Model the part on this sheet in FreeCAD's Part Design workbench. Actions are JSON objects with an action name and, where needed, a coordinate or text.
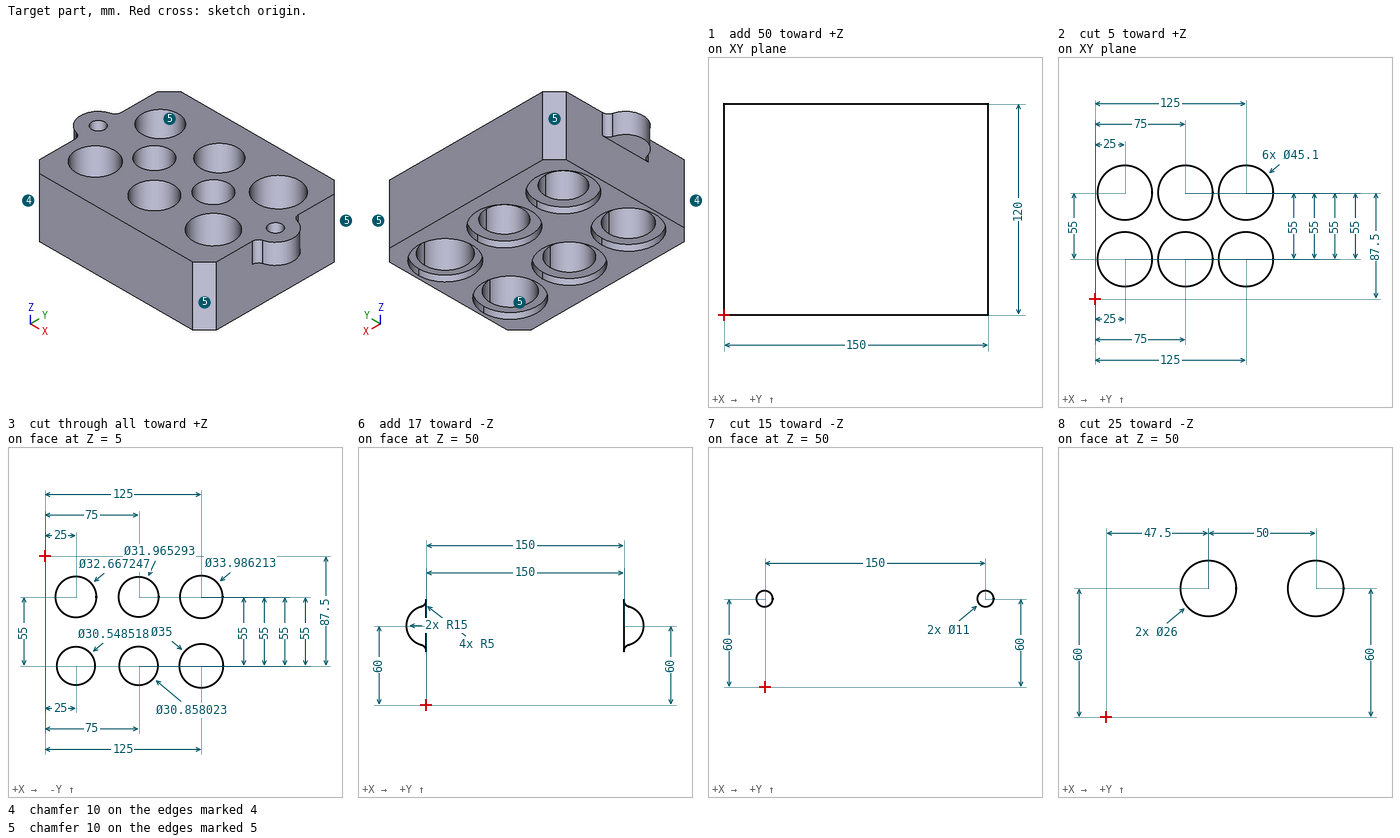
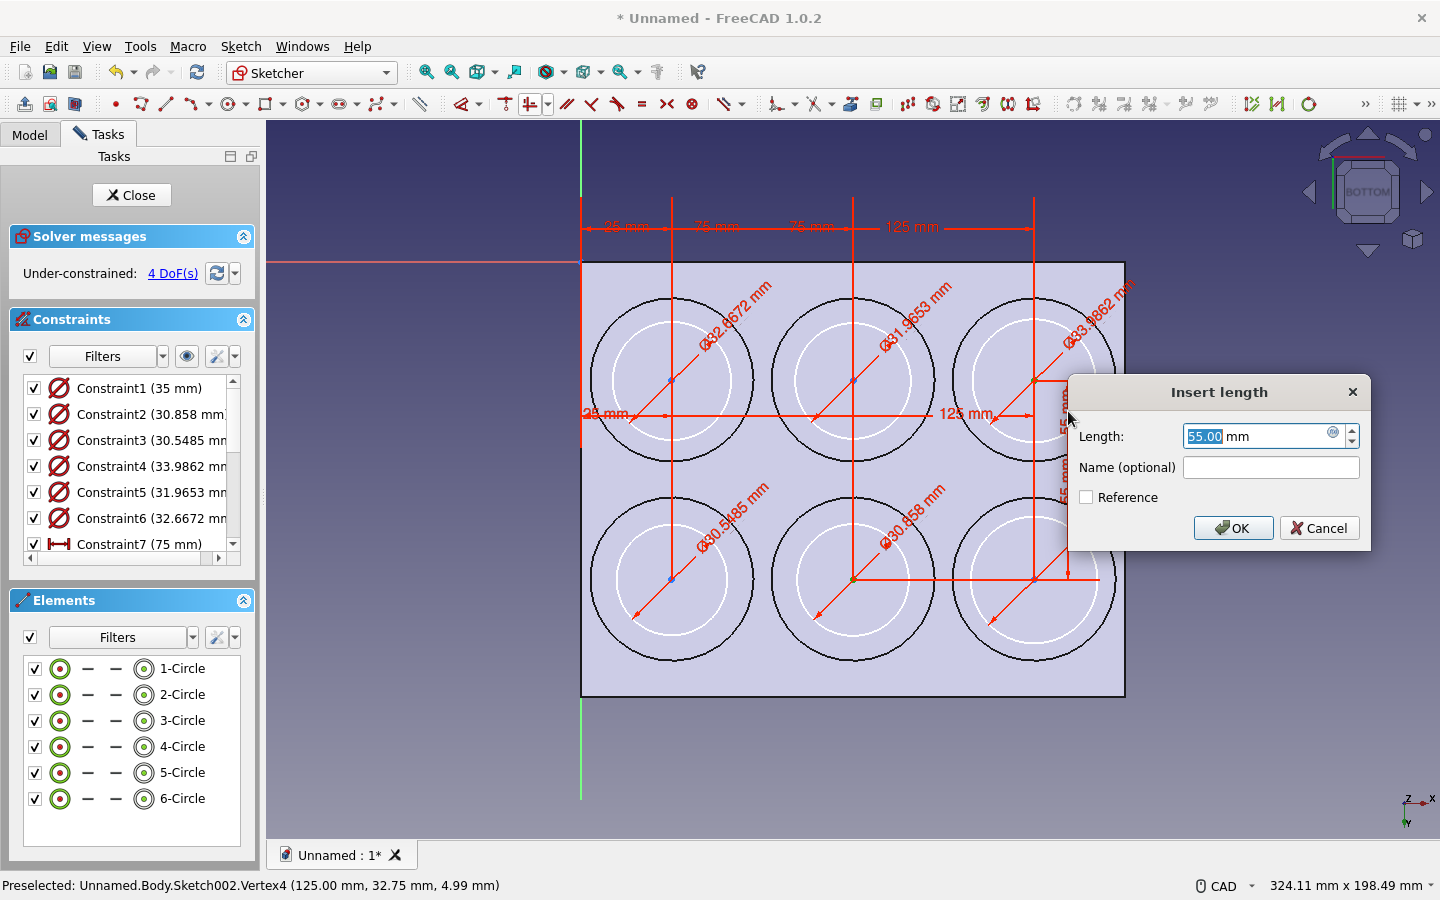
{"action": "type", "text": "55"}
{"action": "key", "text": "Return"}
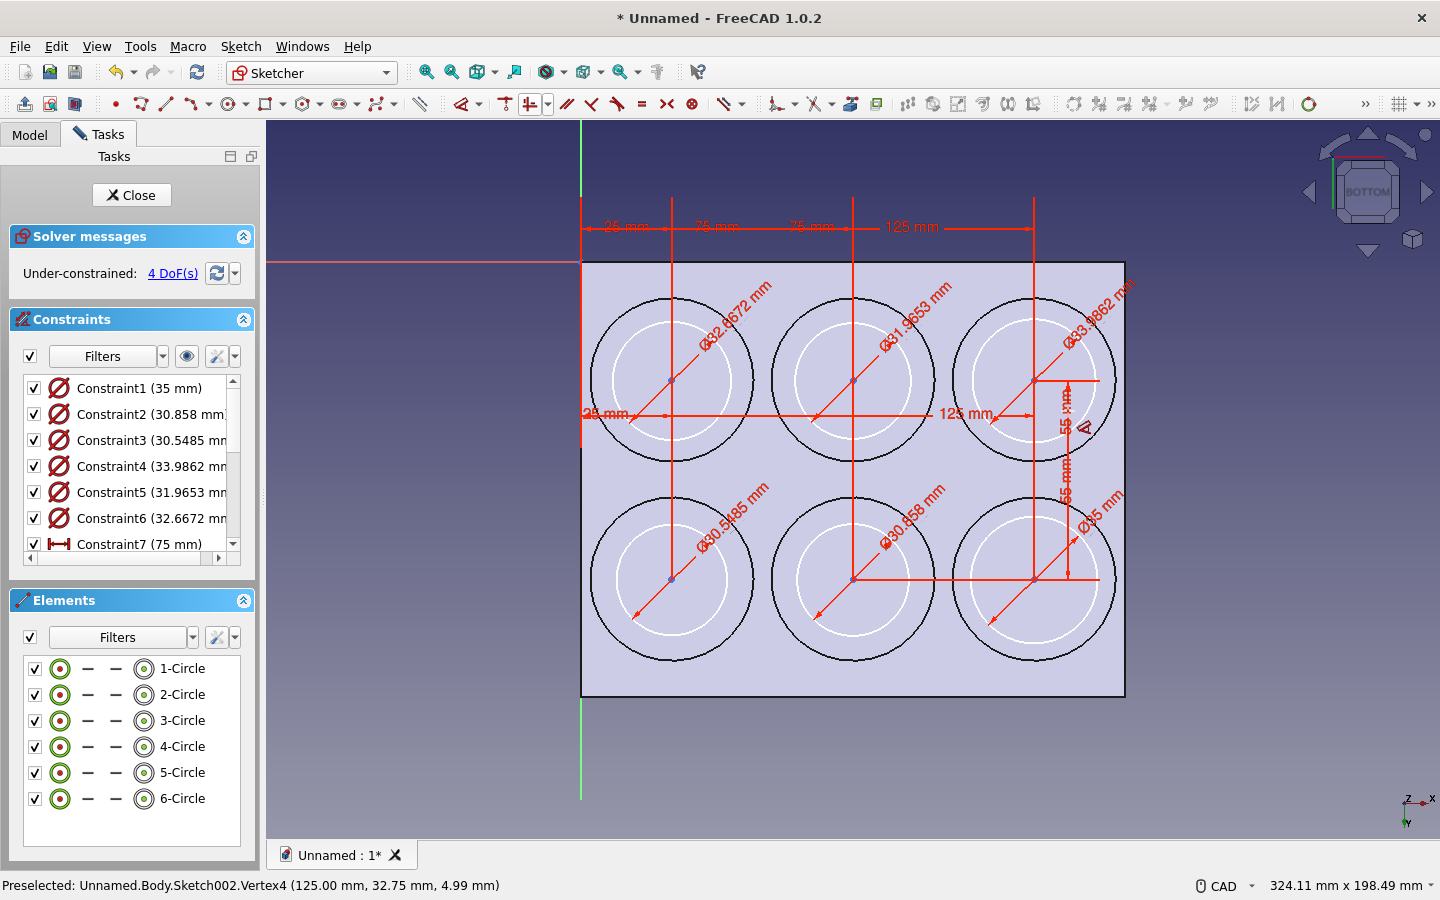
{"action": "left_click", "coordinate": [672, 580]}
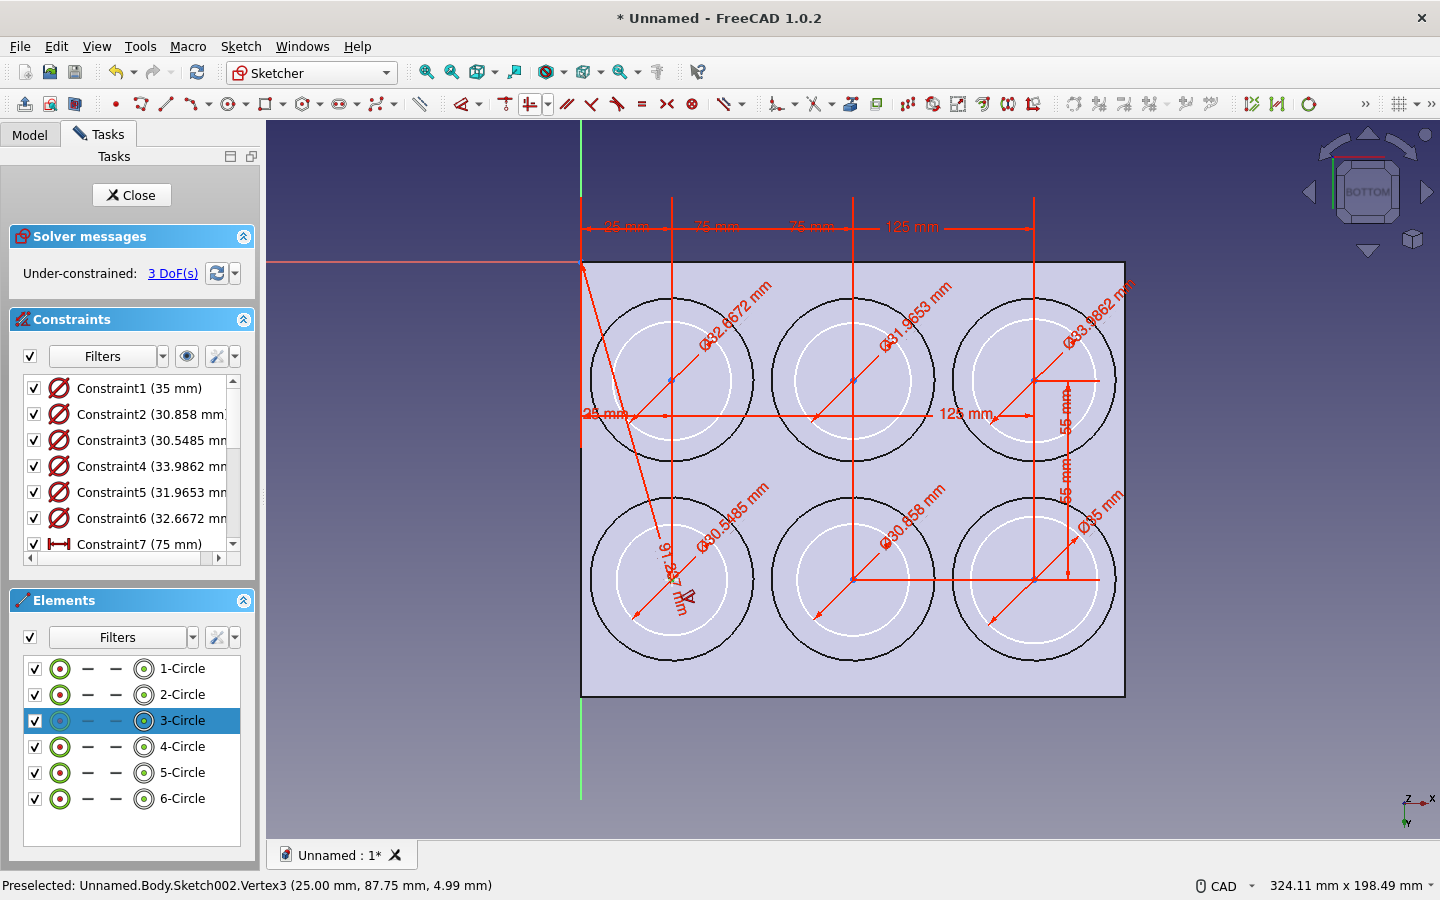
{"action": "left_click", "coordinate": [1034, 381]}
{"action": "left_click", "coordinate": [1068, 550]}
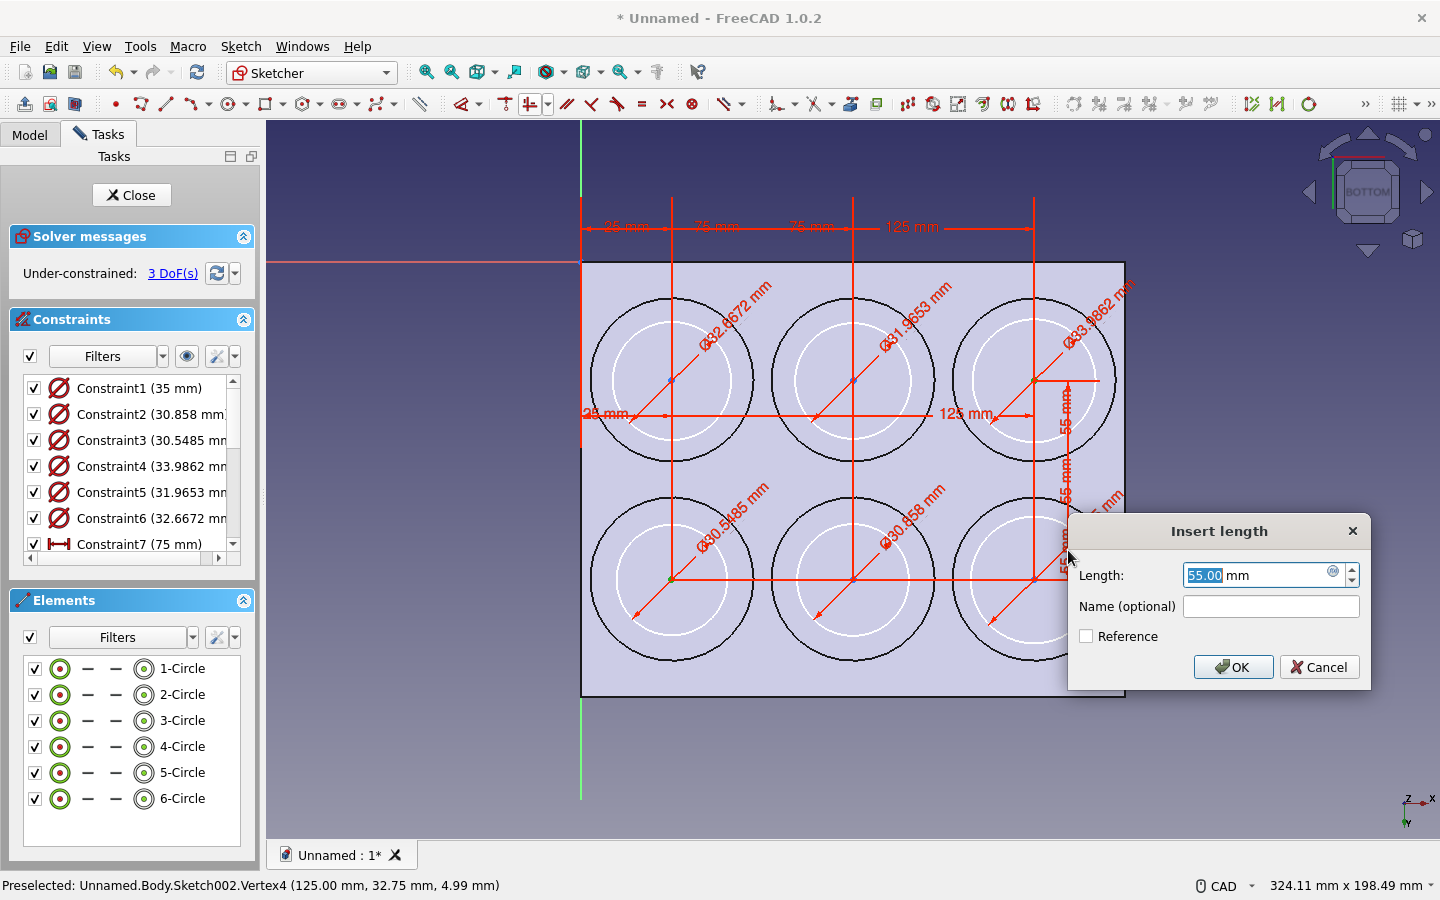
{"action": "type", "text": "55"}
{"action": "key", "text": "Return"}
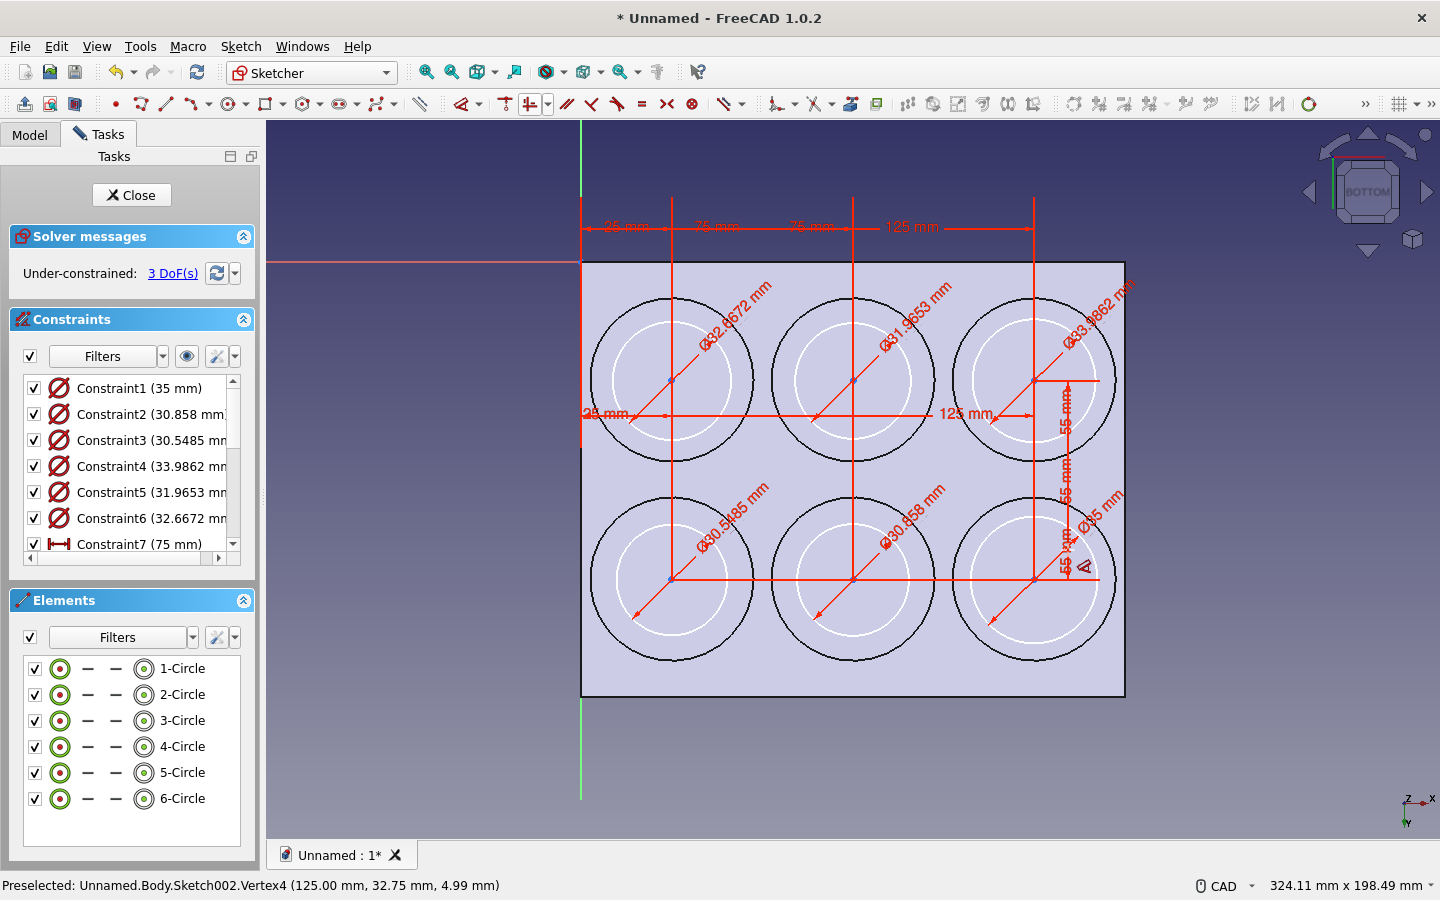
{"action": "left_click", "coordinate": [853, 580]}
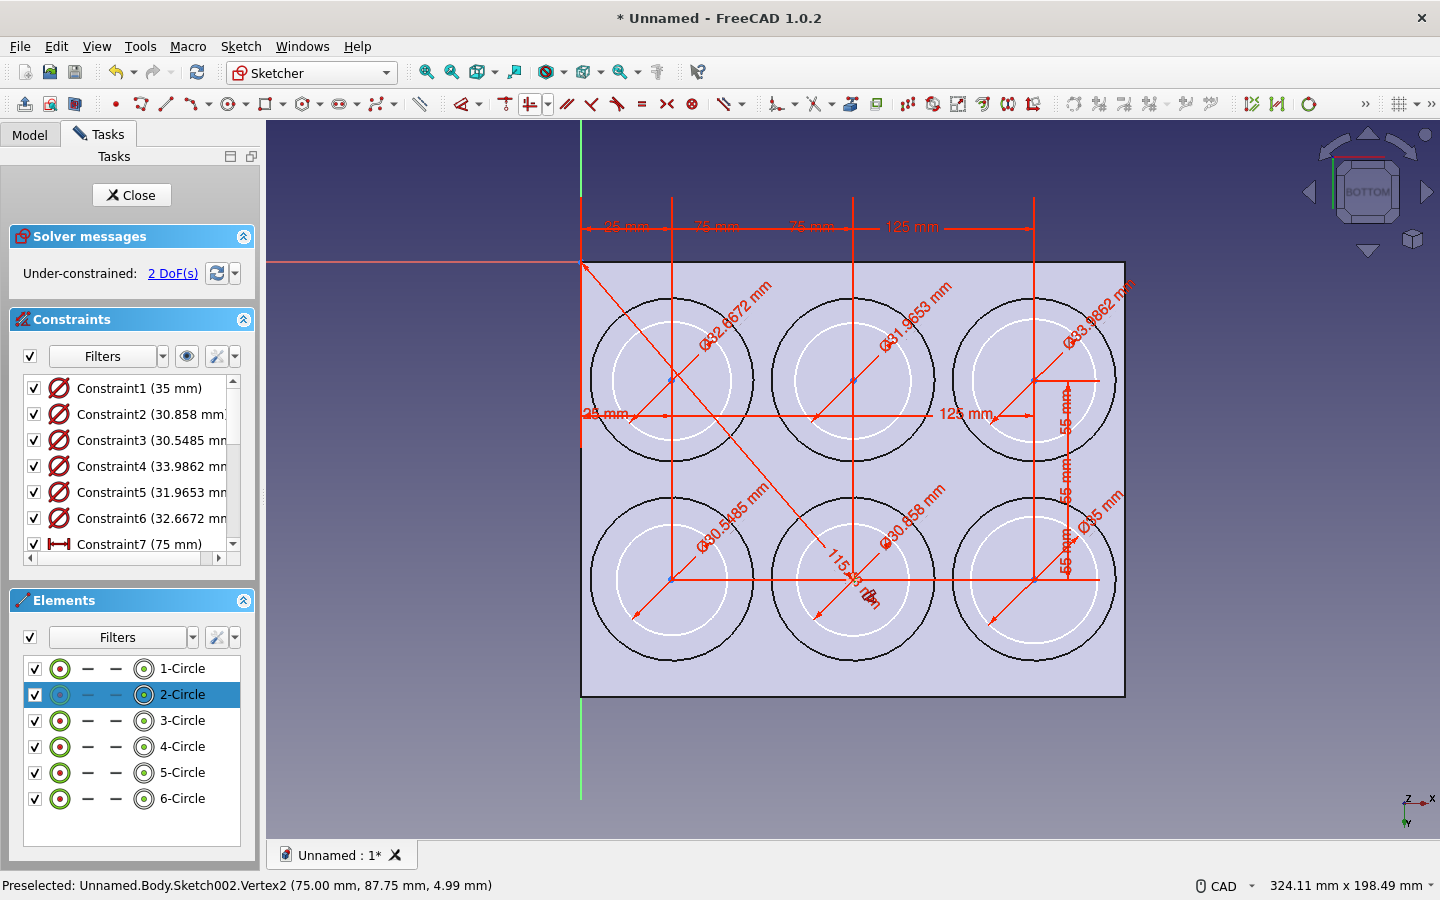
{"action": "left_click", "coordinate": [853, 381]}
{"action": "left_click", "coordinate": [887, 480]}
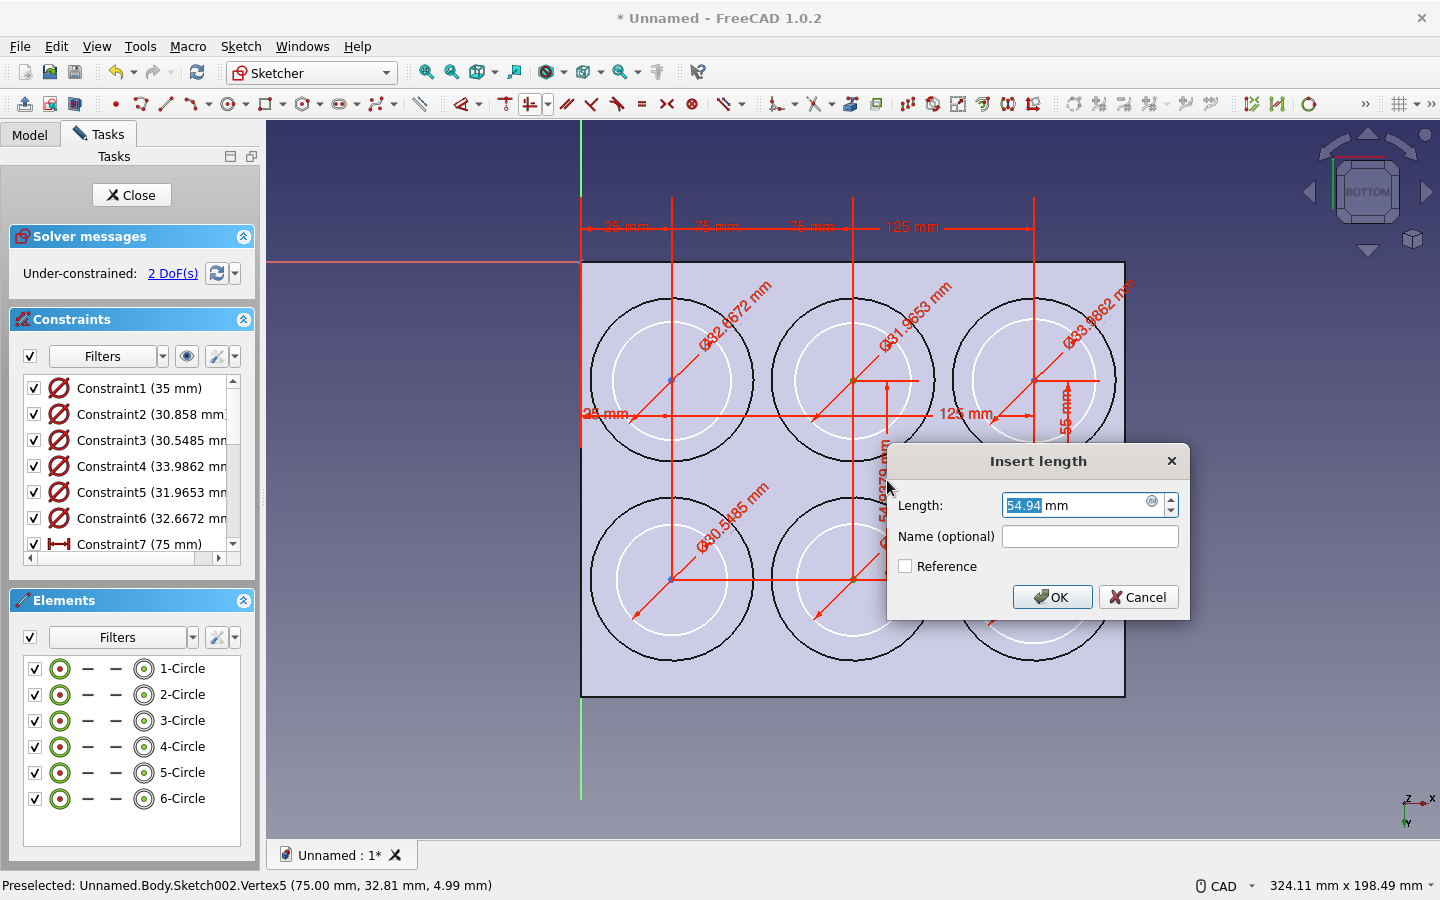
{"action": "type", "text": "55"}
{"action": "key", "text": "Return"}